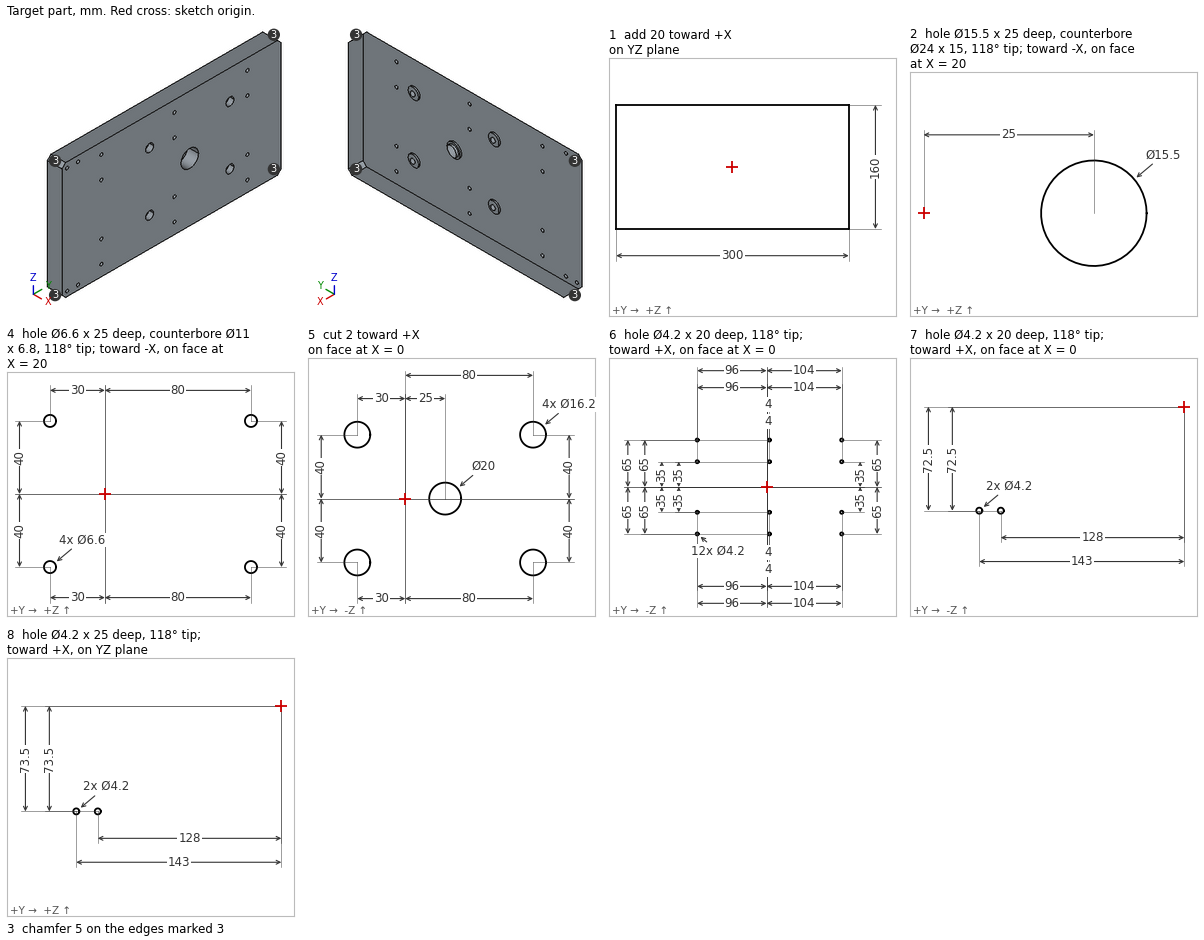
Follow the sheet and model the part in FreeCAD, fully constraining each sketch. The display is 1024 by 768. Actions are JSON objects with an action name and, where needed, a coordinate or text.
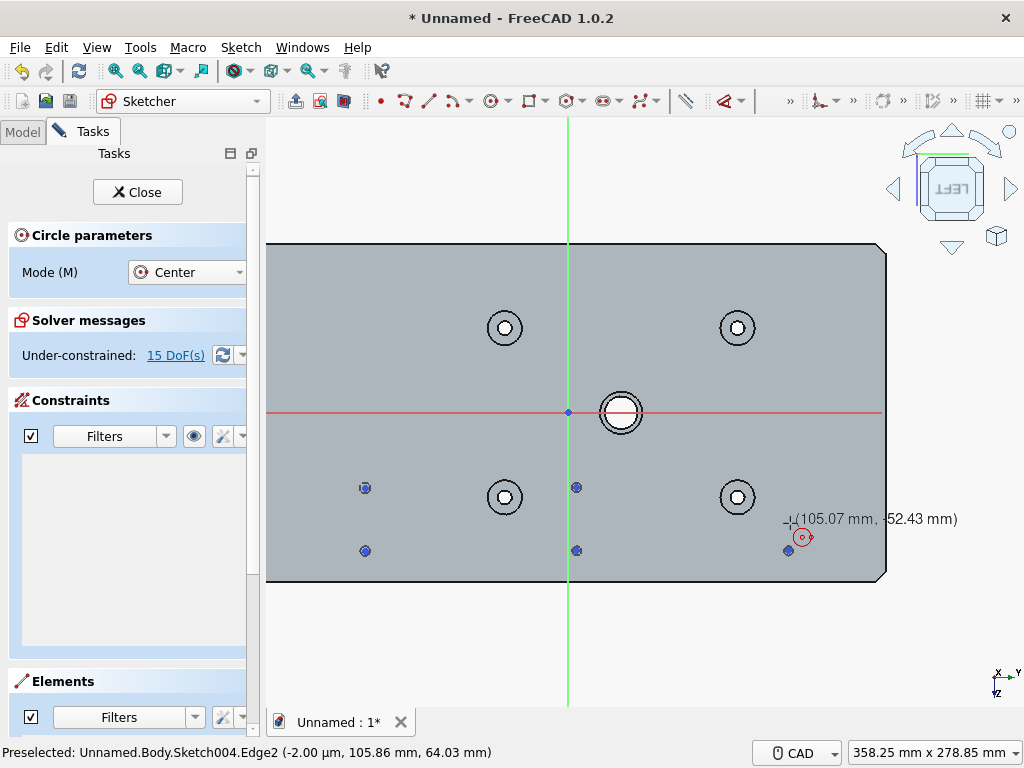
{"action": "left_click", "coordinate": [788, 487]}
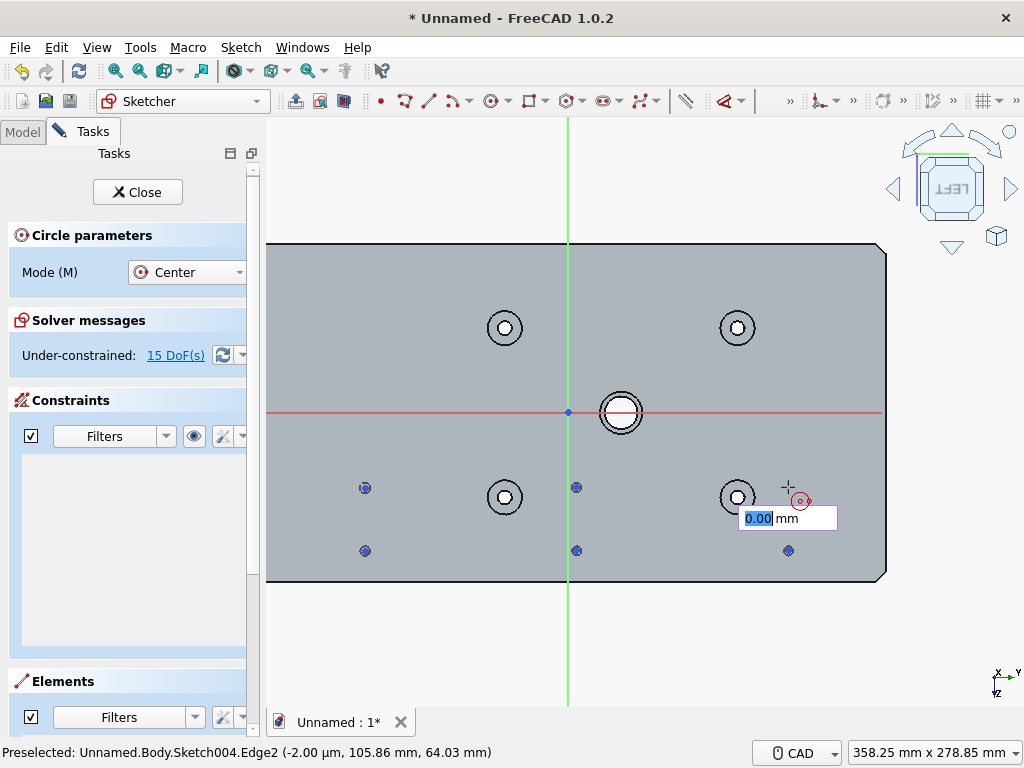
{"action": "scroll", "coordinate": [791, 484], "scroll_direction": "up", "scroll_amount": 7}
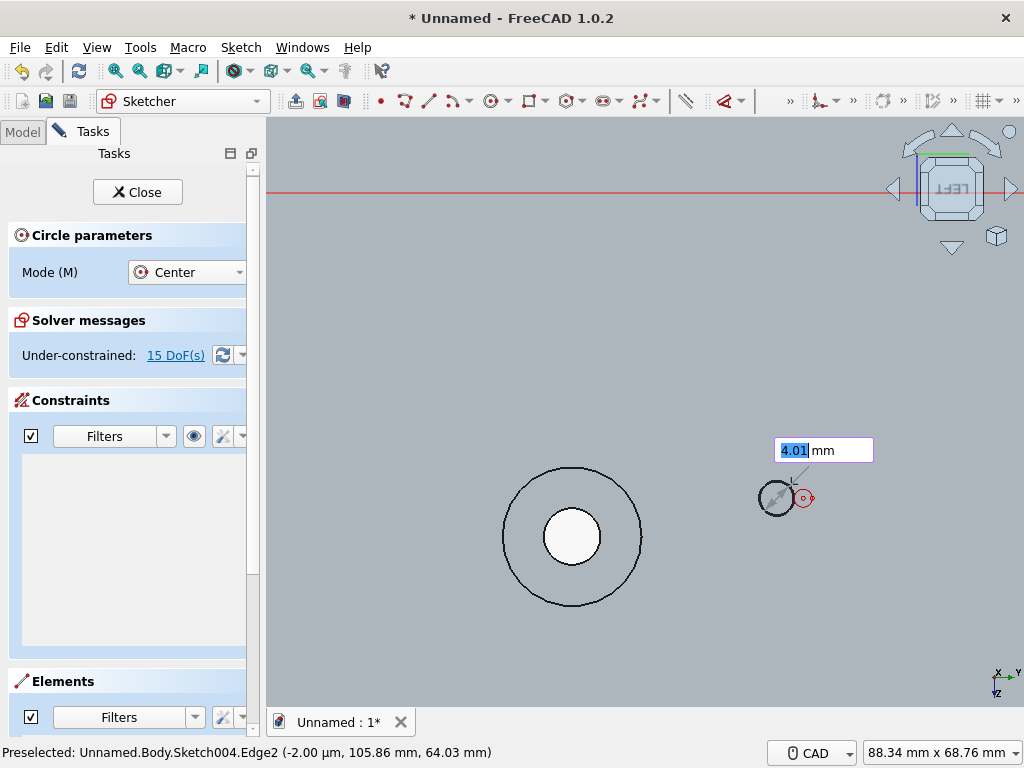
{"action": "left_click", "coordinate": [791, 481]}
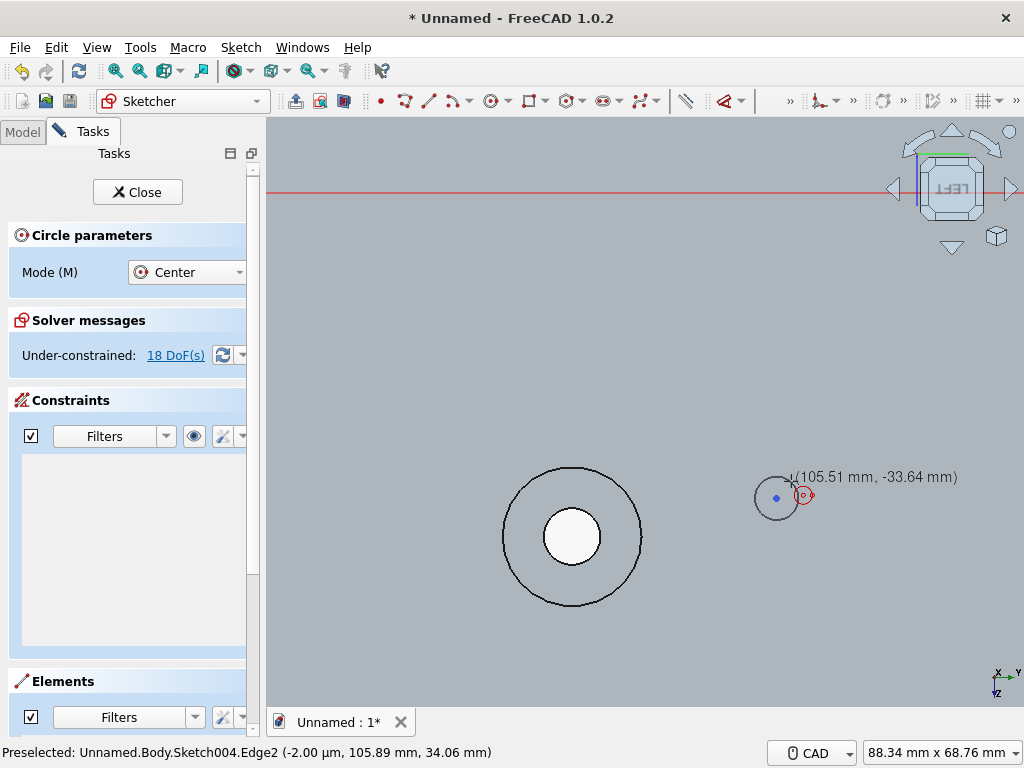
{"action": "scroll", "coordinate": [791, 484], "scroll_direction": "down", "scroll_amount": 7}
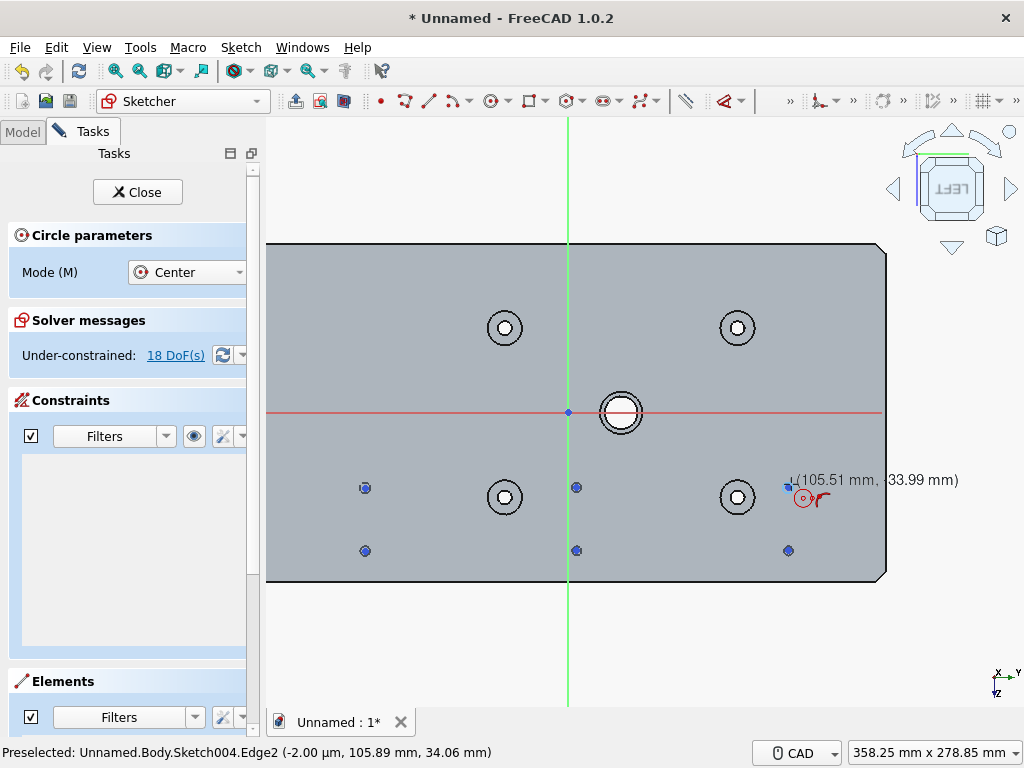
{"action": "scroll", "coordinate": [788, 339], "scroll_direction": "up", "scroll_amount": 9}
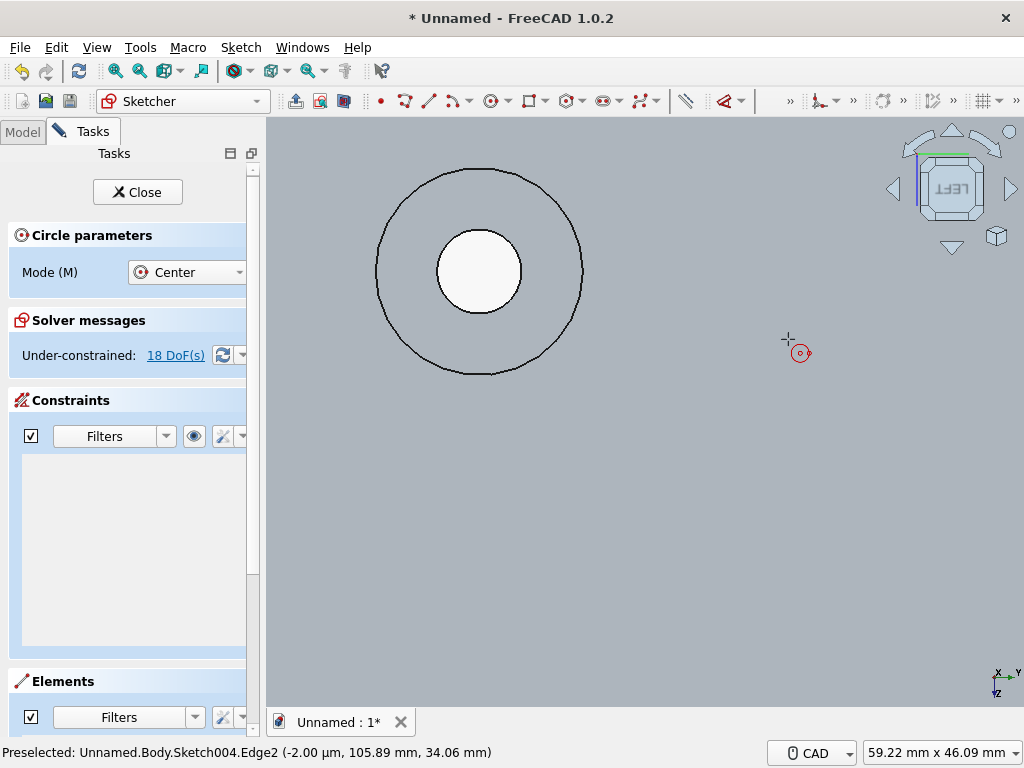
{"action": "scroll", "coordinate": [788, 338], "scroll_direction": "down", "scroll_amount": 9}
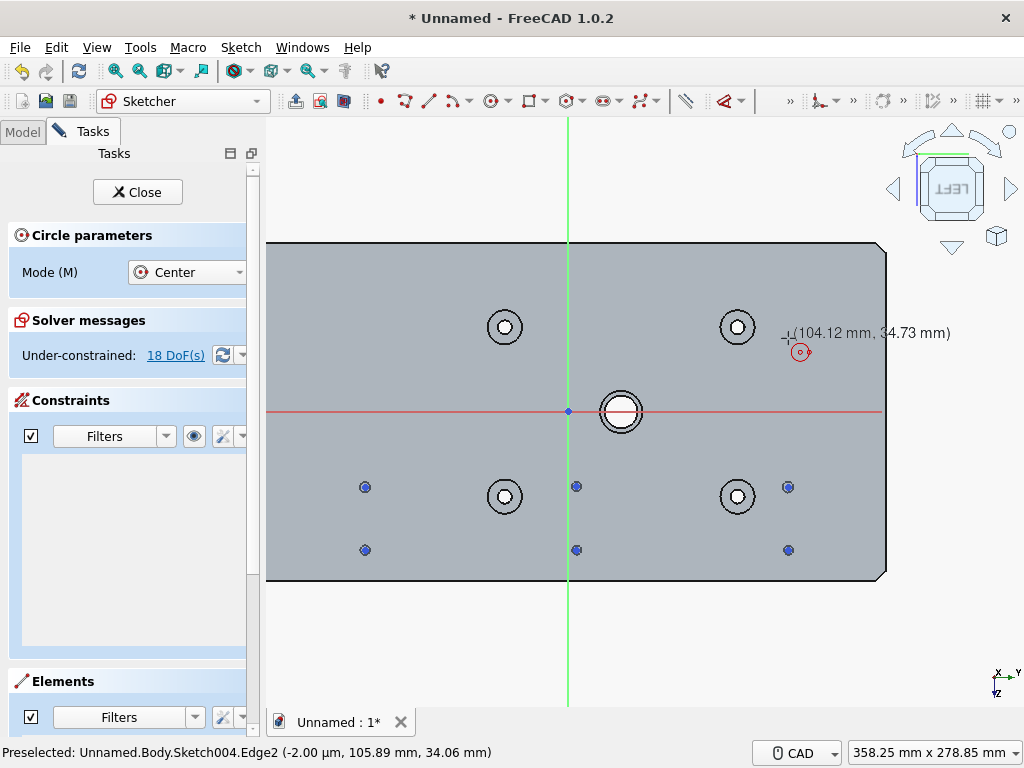
{"action": "left_click", "coordinate": [788, 338]}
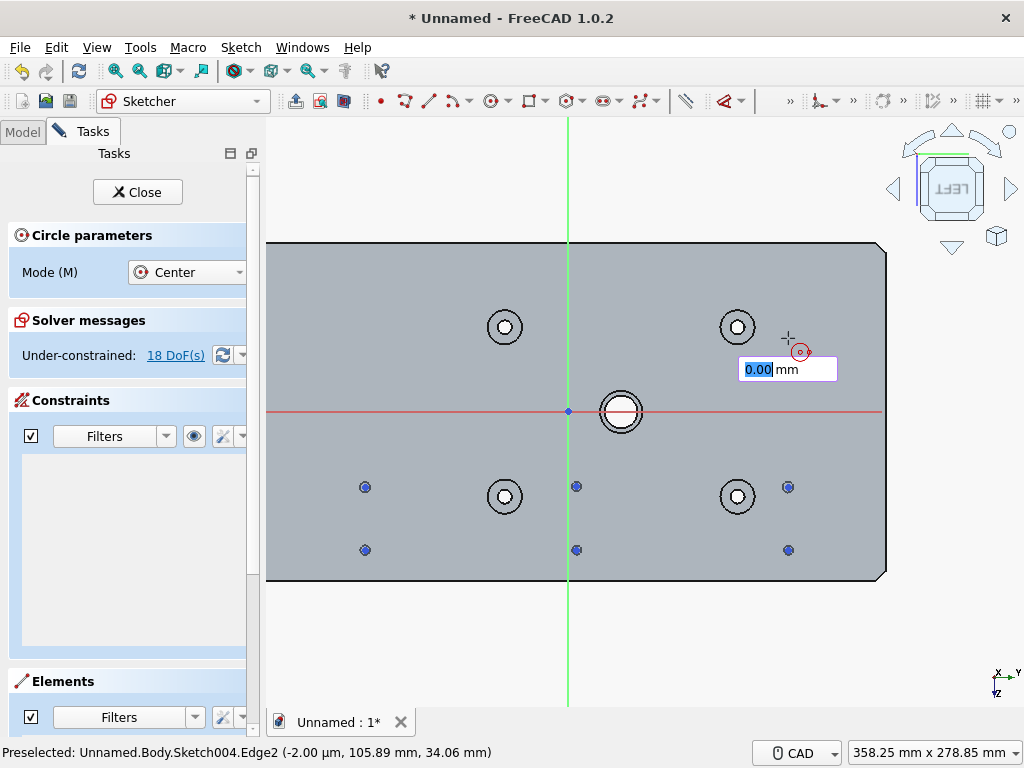
{"action": "scroll", "coordinate": [791, 335], "scroll_direction": "up", "scroll_amount": 7}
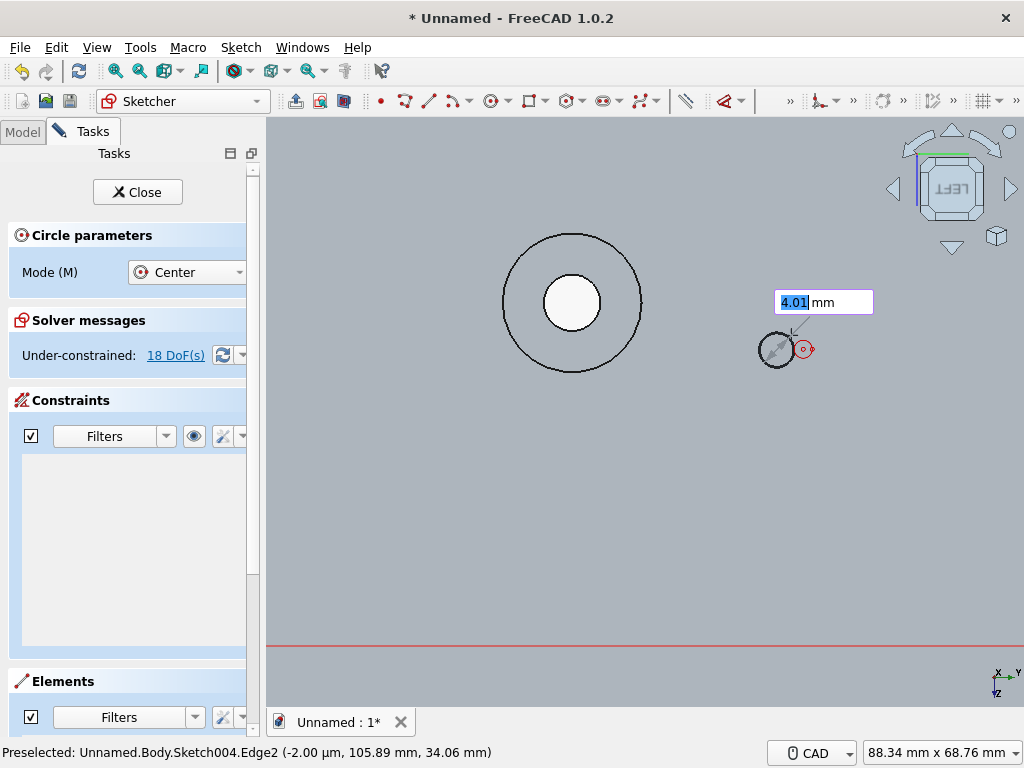
{"action": "left_click", "coordinate": [791, 333]}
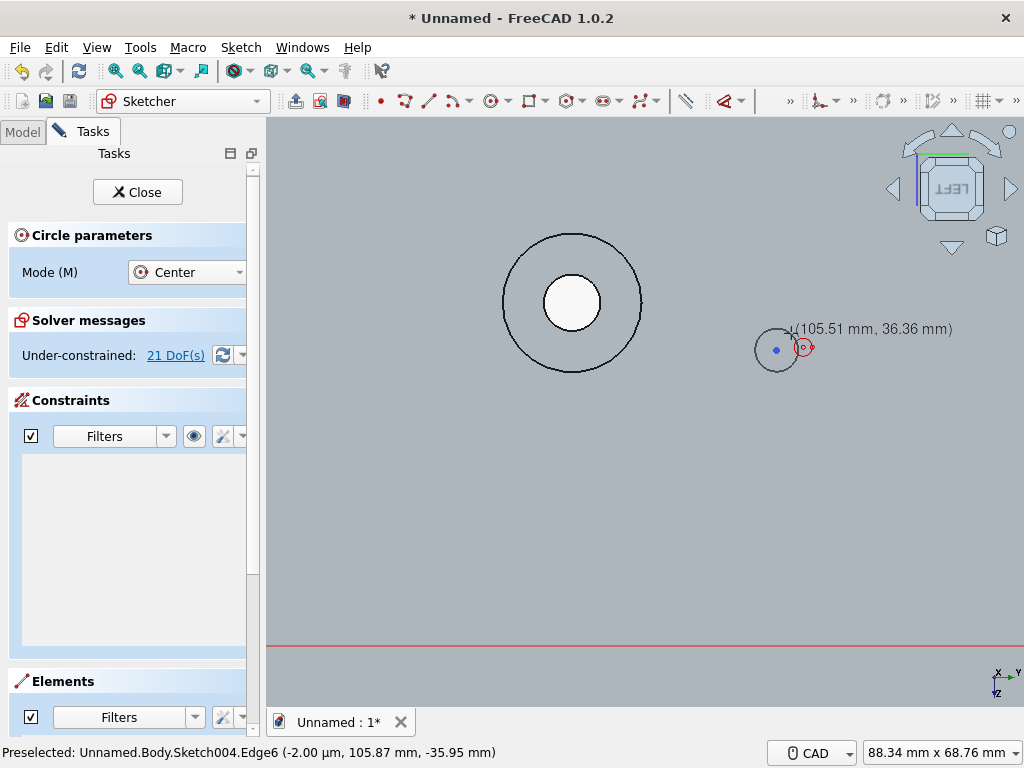
{"action": "scroll", "coordinate": [791, 335], "scroll_direction": "down", "scroll_amount": 7}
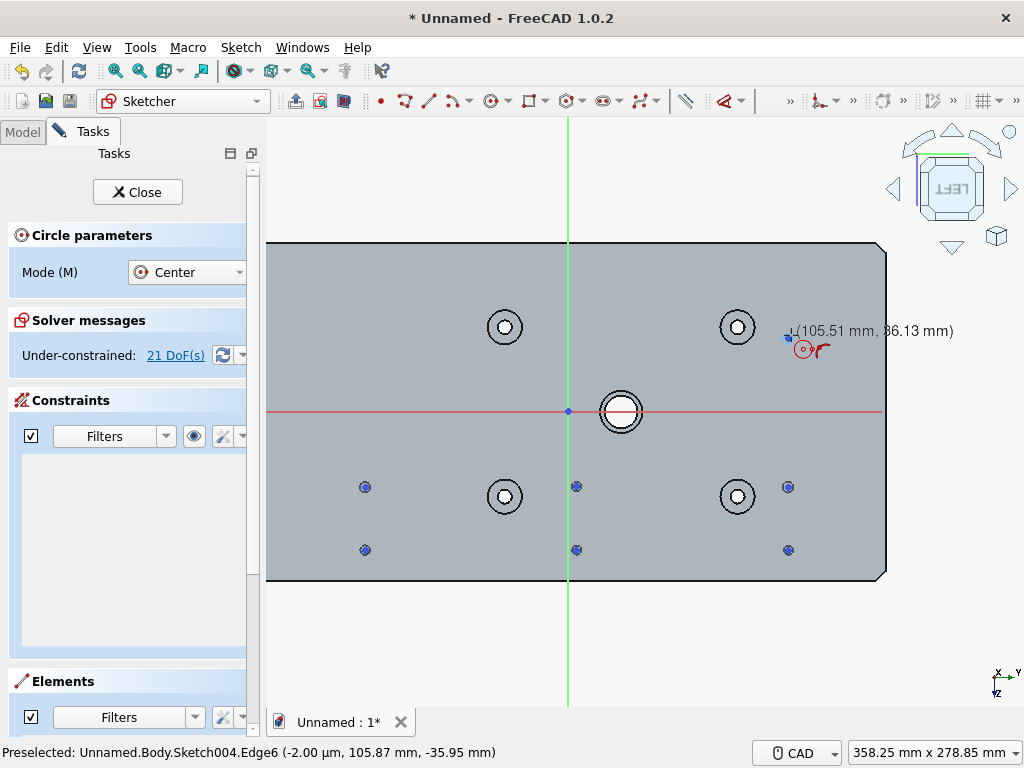
{"action": "scroll", "coordinate": [788, 274], "scroll_direction": "up", "scroll_amount": 9}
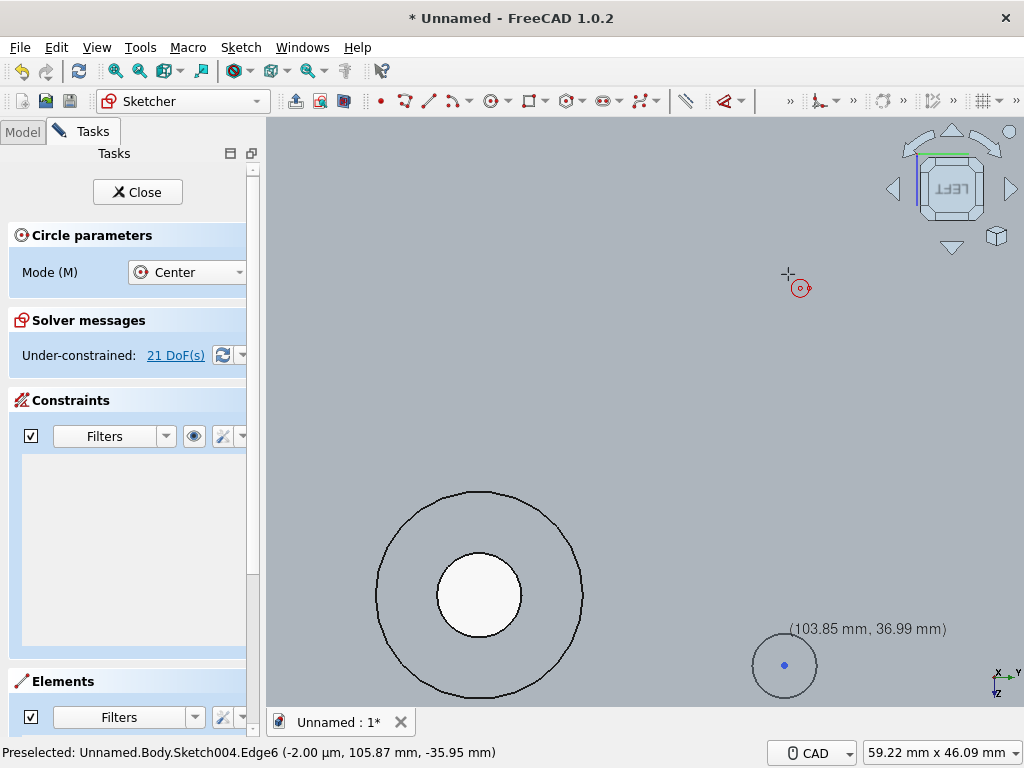
{"action": "scroll", "coordinate": [788, 274], "scroll_direction": "down", "scroll_amount": 9}